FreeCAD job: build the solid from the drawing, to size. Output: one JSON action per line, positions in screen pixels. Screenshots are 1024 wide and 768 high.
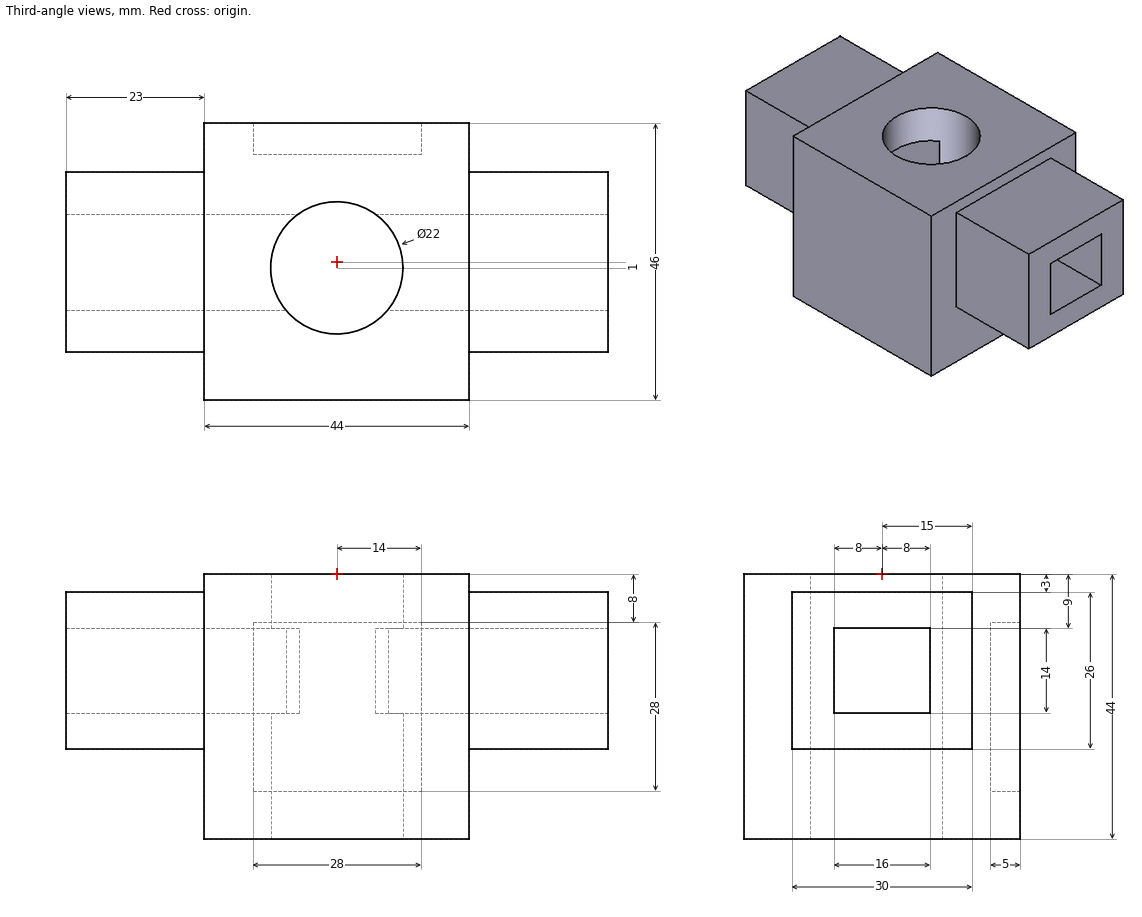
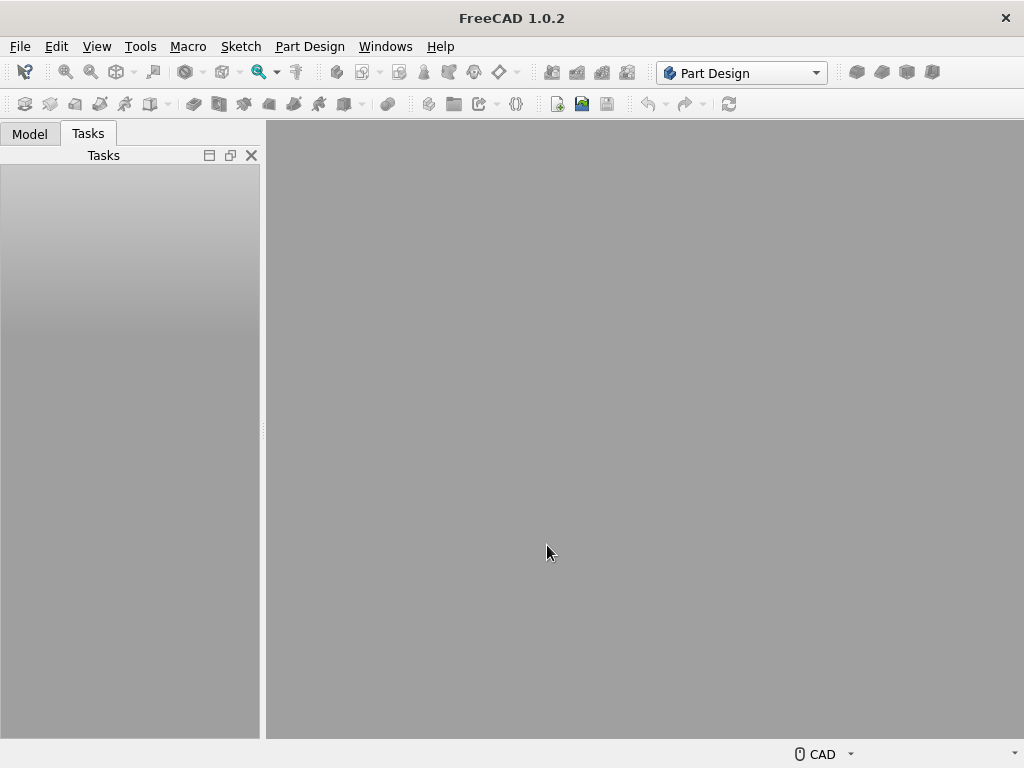
{"action": "key", "text": "ctrl+n"}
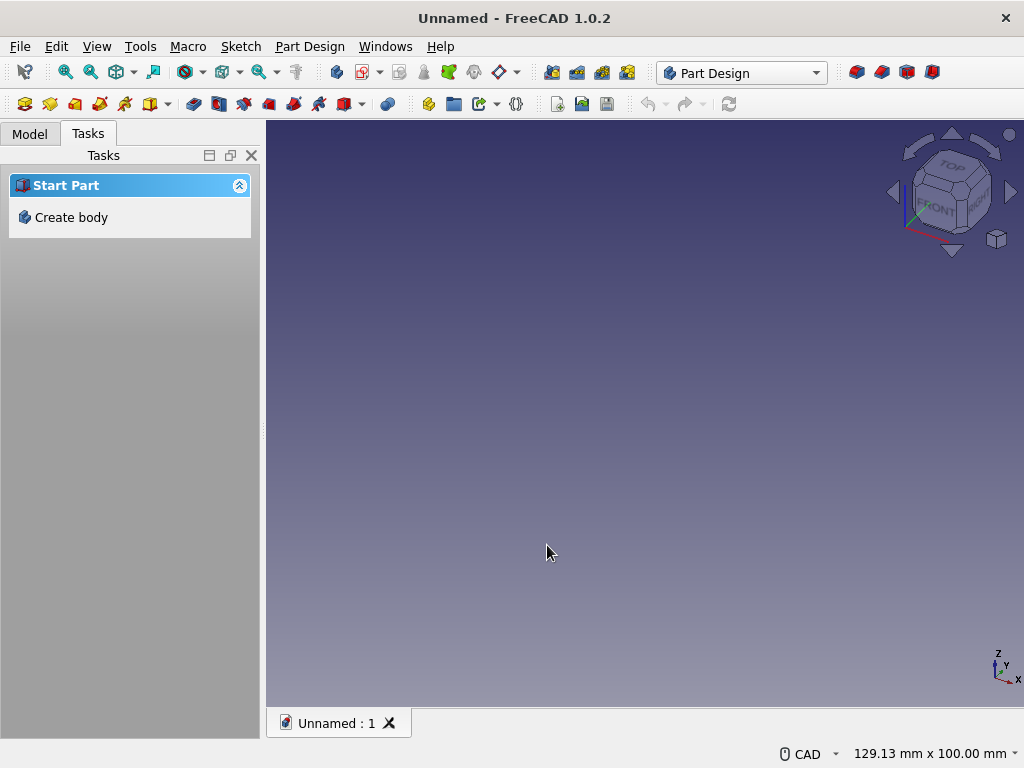
{"action": "left_click", "coordinate": [362, 72]}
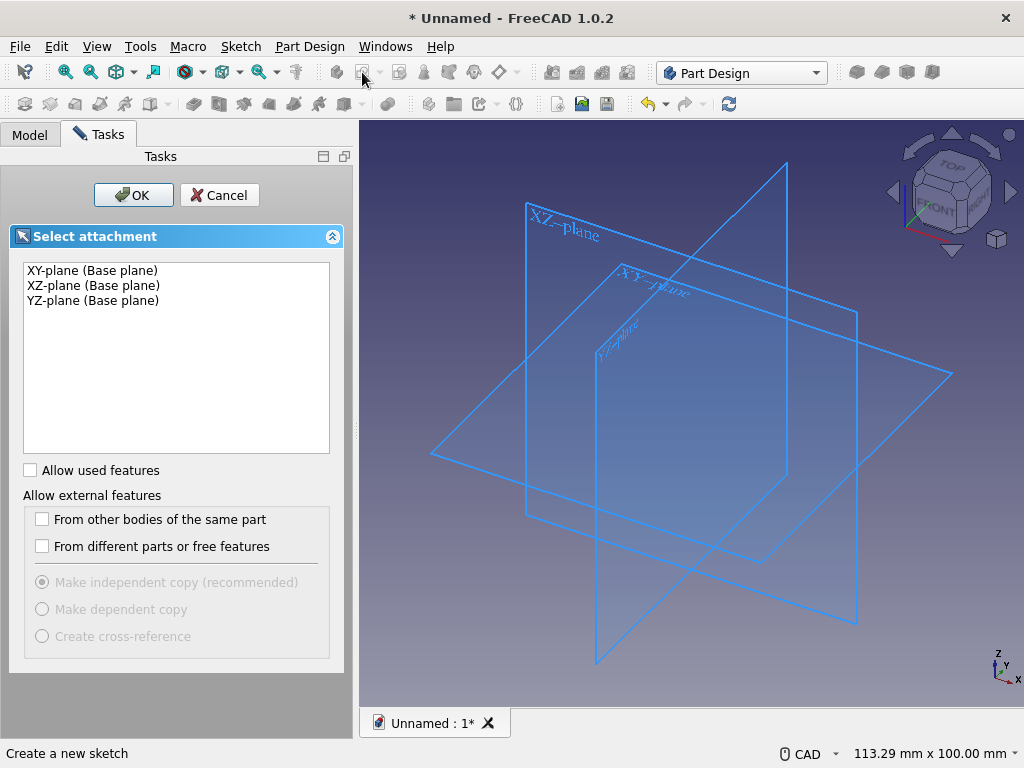
{"action": "left_click", "coordinate": [84, 270]}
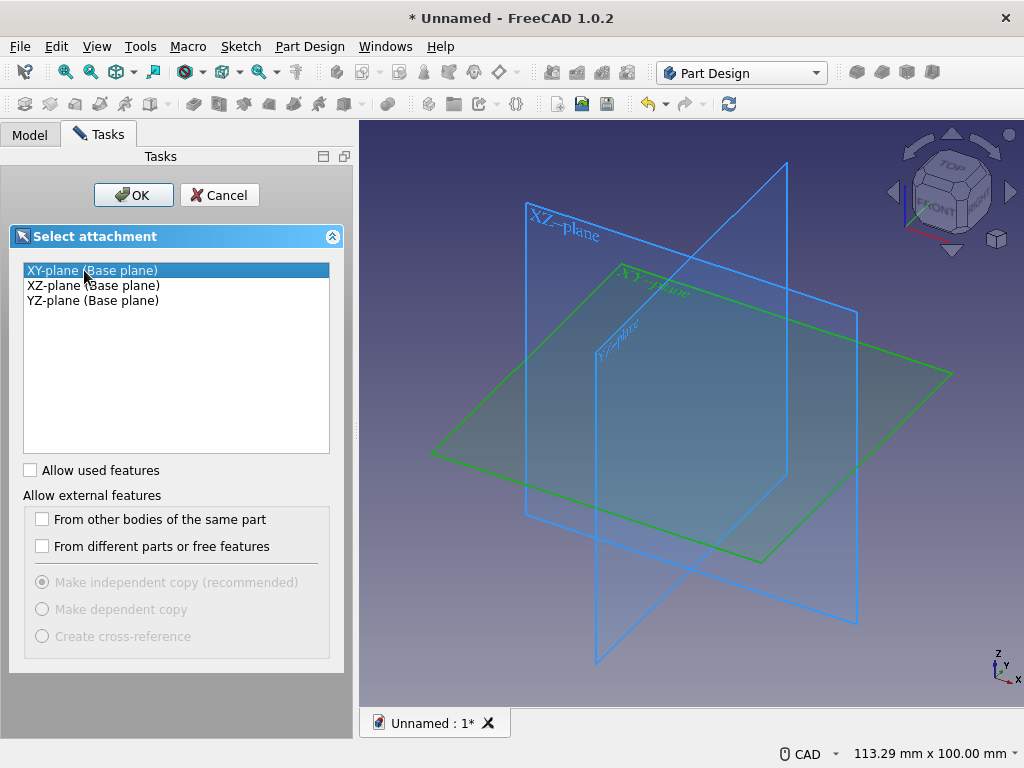
{"action": "left_click", "coordinate": [134, 195]}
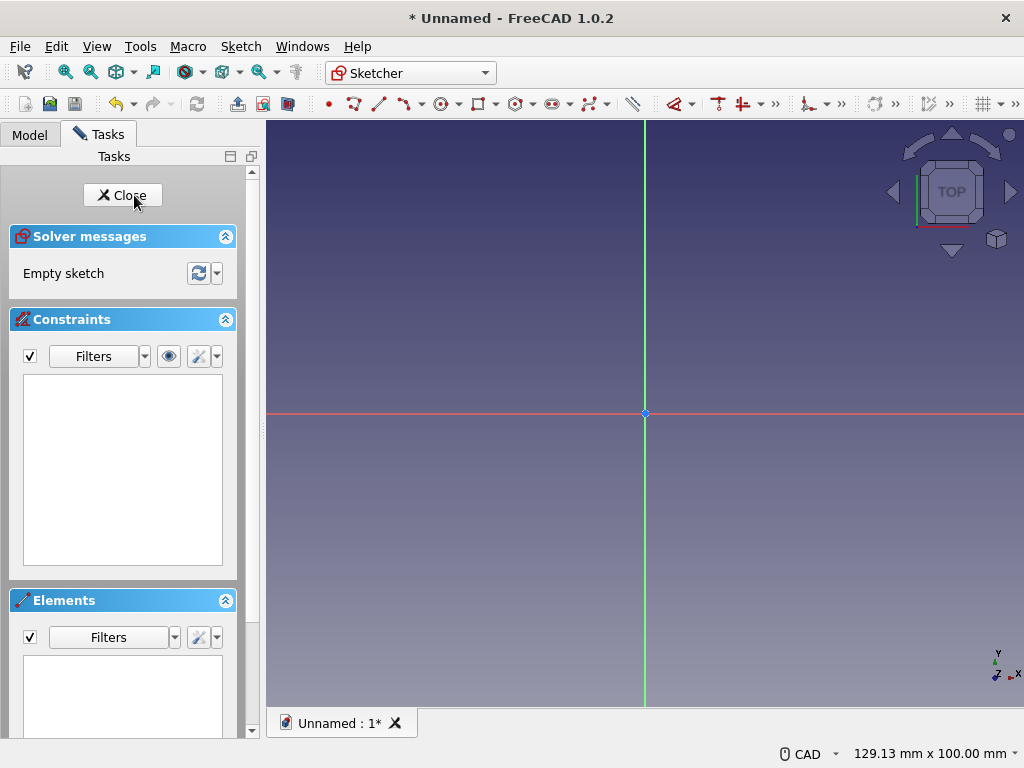
{"action": "scroll", "coordinate": [784, 413], "scroll_direction": "up", "scroll_amount": 2}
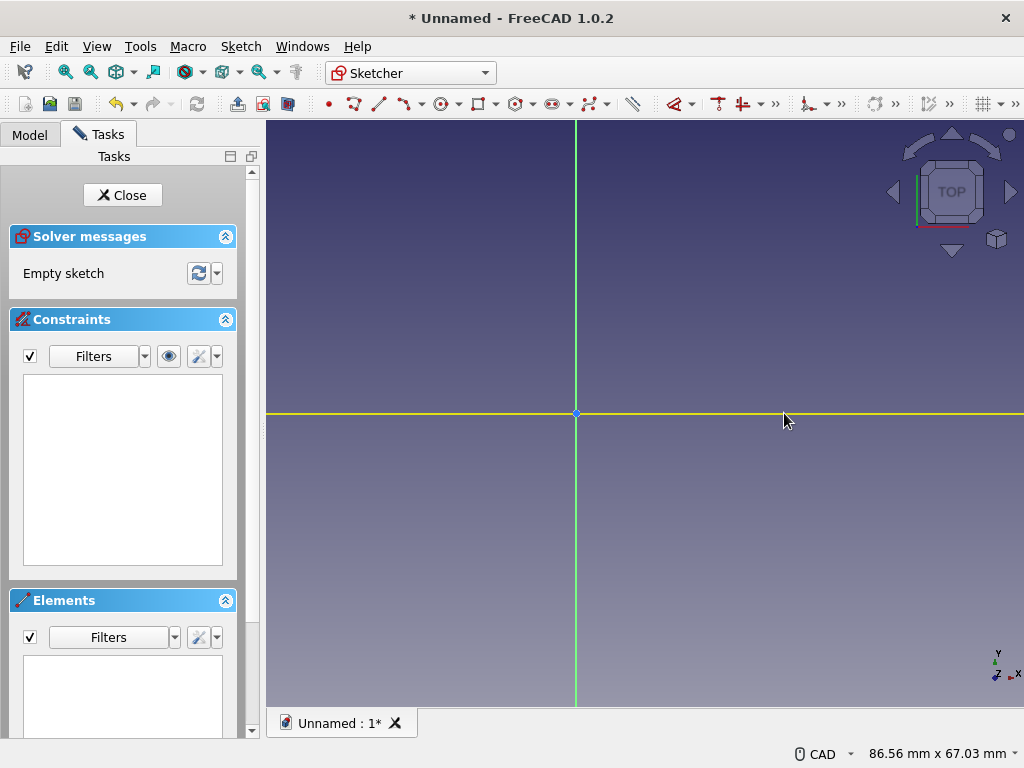
{"action": "key", "text": "g v"}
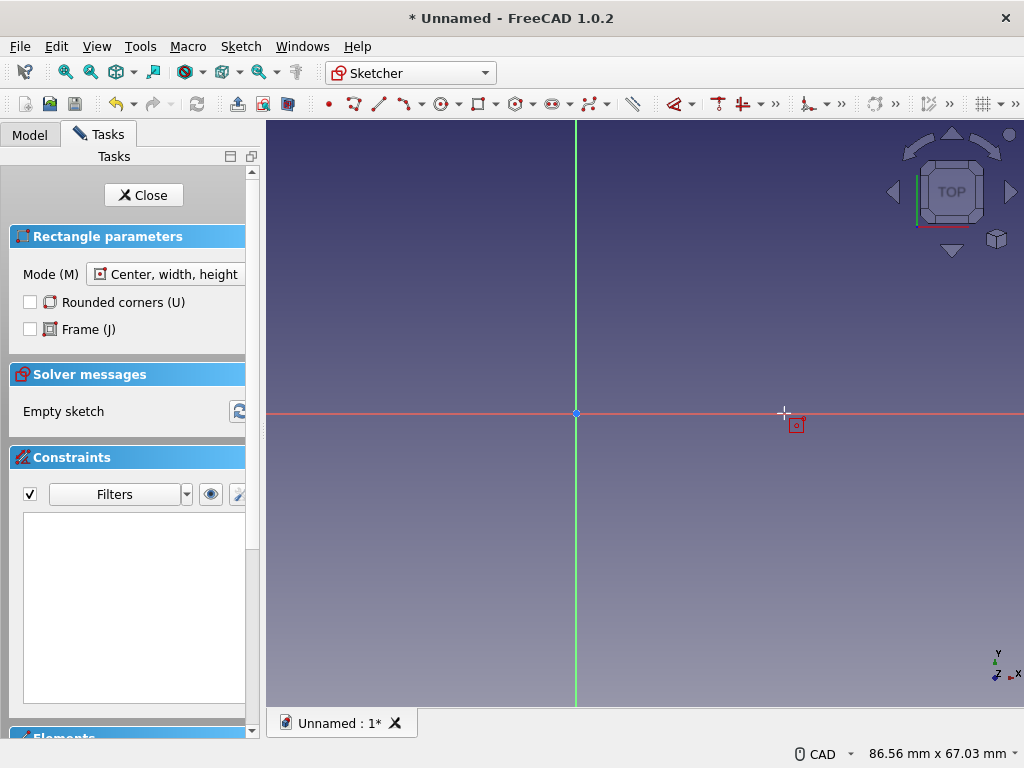
{"action": "left_click", "coordinate": [576, 414]}
{"action": "left_click", "coordinate": [769, 212]}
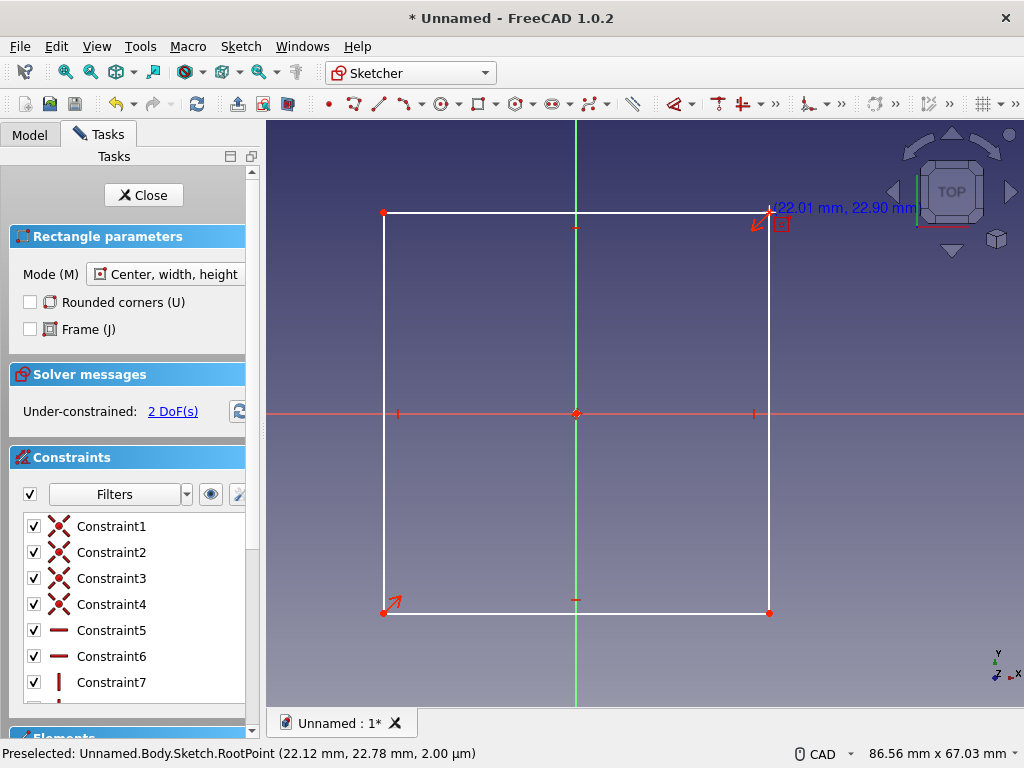
{"action": "key", "text": "g c"}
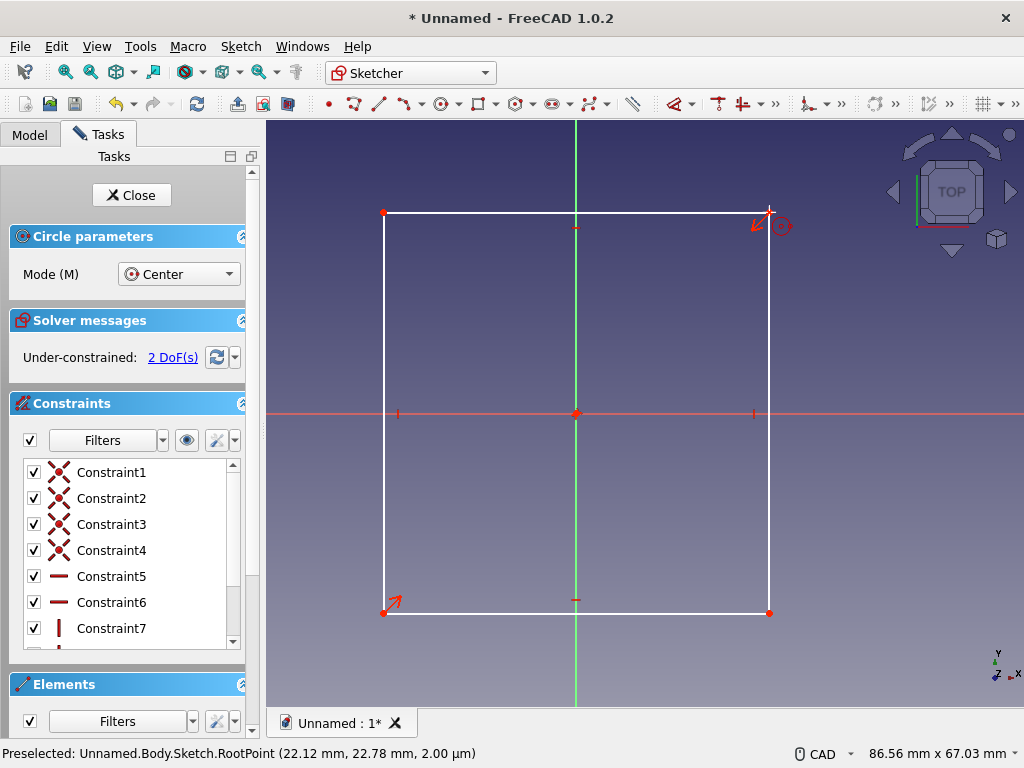
{"action": "scroll", "coordinate": [576, 422], "scroll_direction": "up", "scroll_amount": 3}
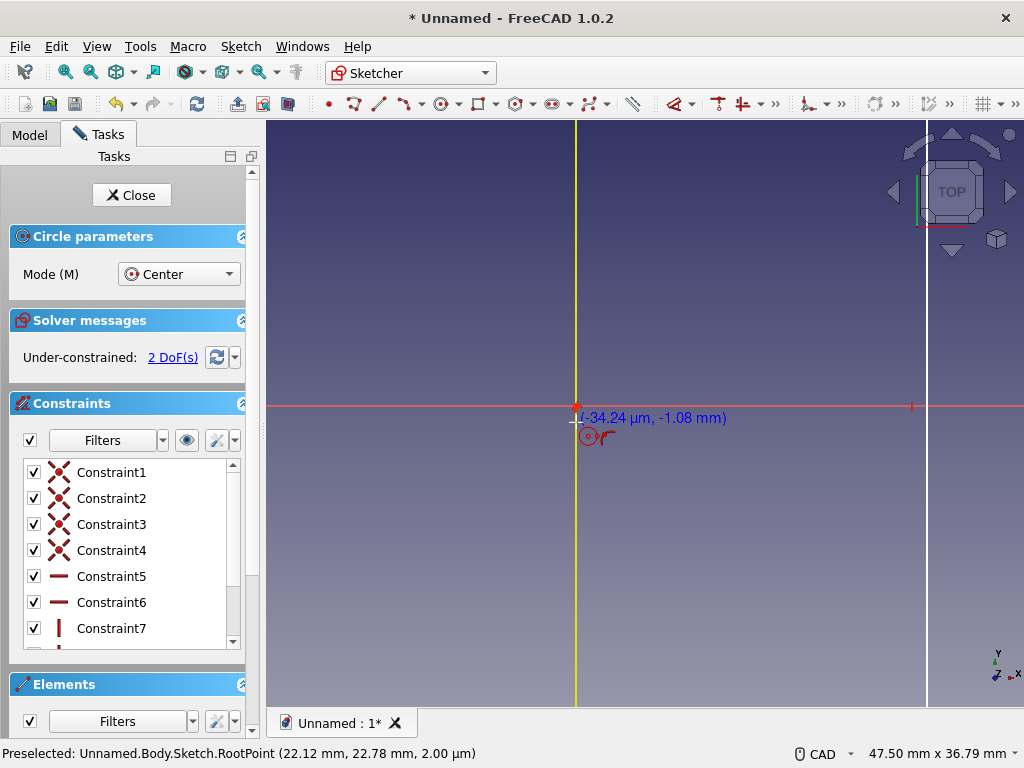
{"action": "left_click", "coordinate": [576, 422]}
{"action": "left_click", "coordinate": [700, 298]}
{"action": "key", "text": "Escape"}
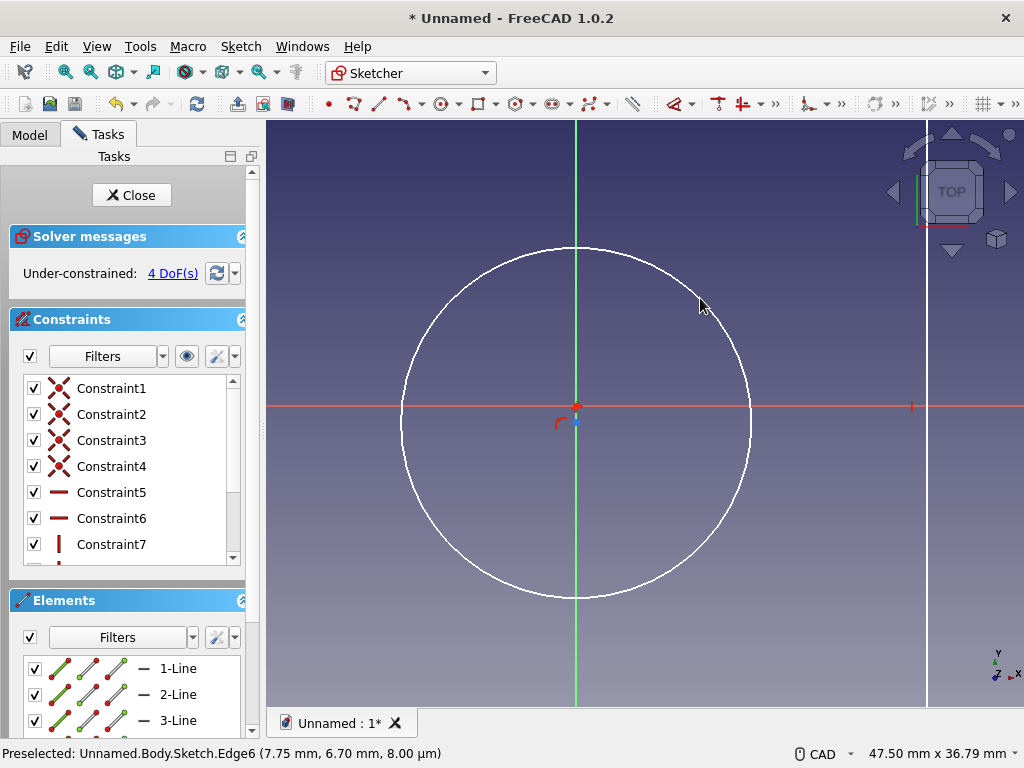
{"action": "left_click", "coordinate": [700, 299]}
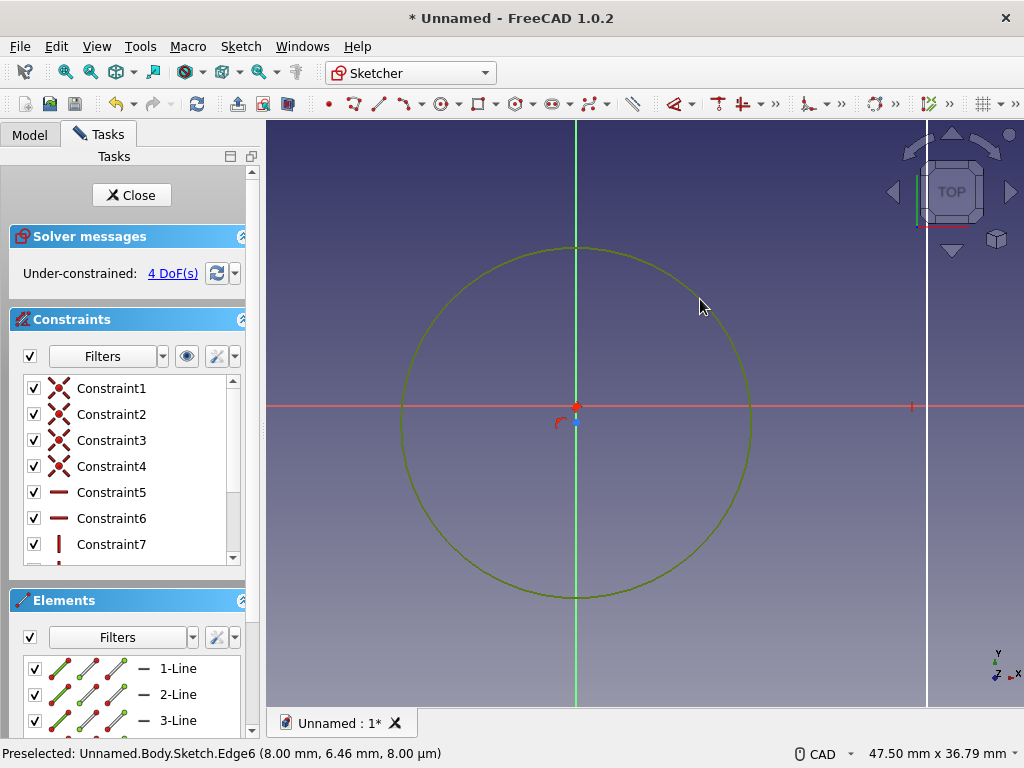
{"action": "key", "text": "k o"}